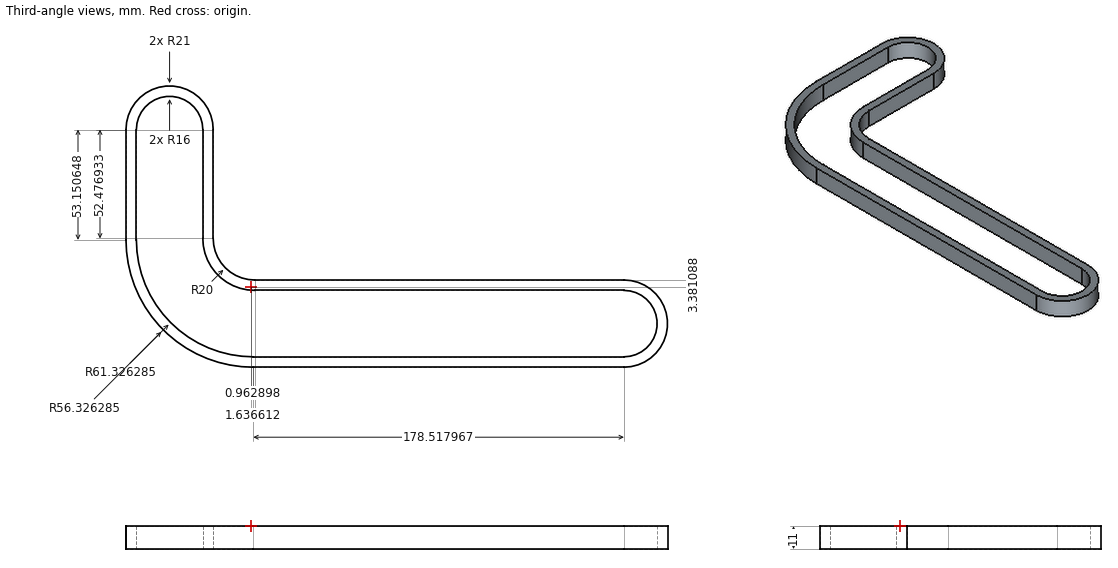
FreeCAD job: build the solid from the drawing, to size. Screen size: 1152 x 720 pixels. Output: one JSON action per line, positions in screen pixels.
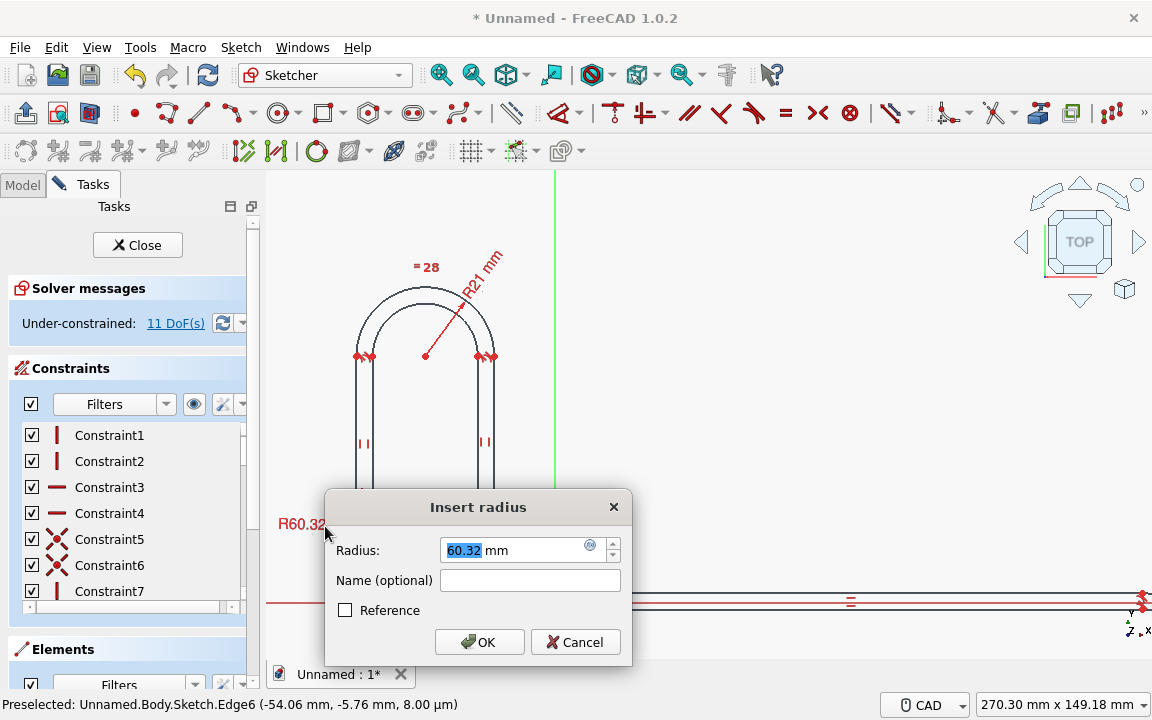
{"action": "type", "text": "61.326285"}
{"action": "key", "text": "Return"}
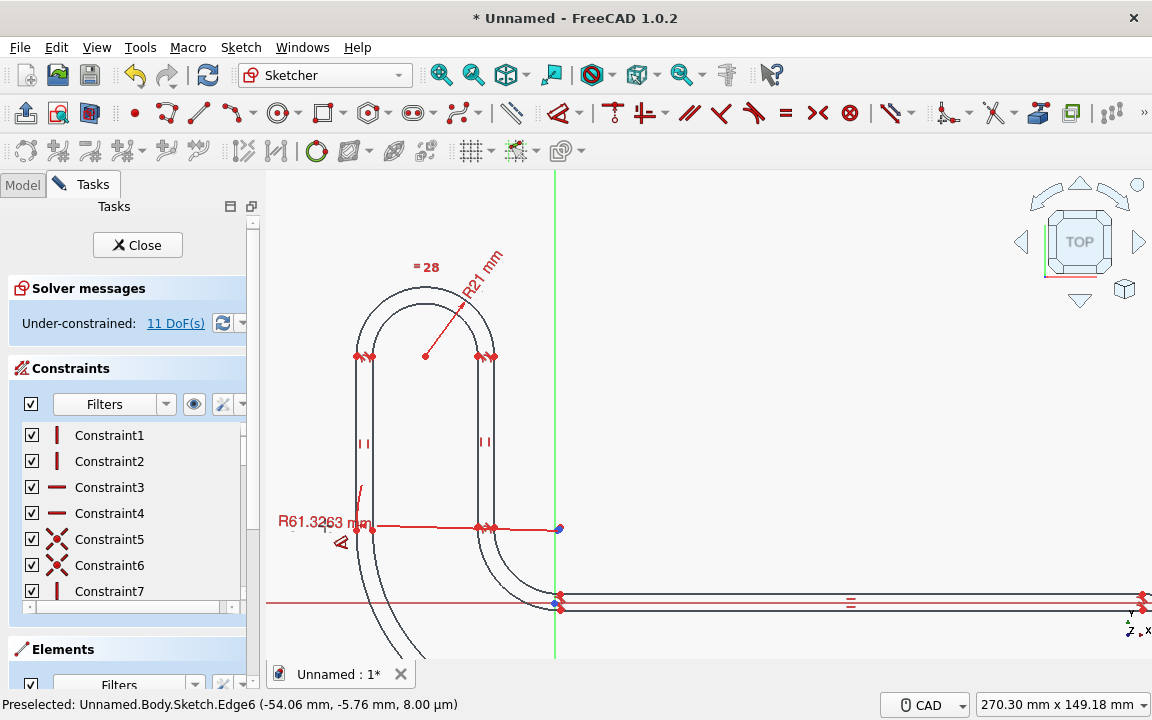
{"action": "left_click", "coordinate": [501, 558]}
{"action": "left_click", "coordinate": [473, 573]}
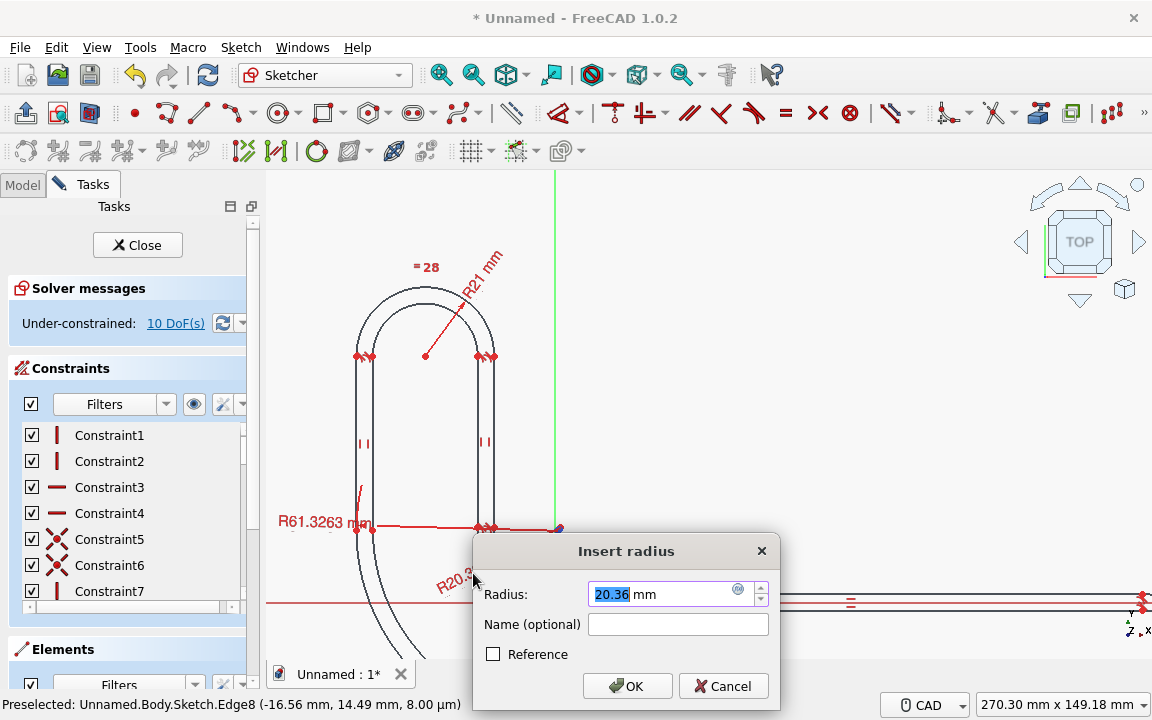
{"action": "type", "text": "20"}
{"action": "key", "text": "Return"}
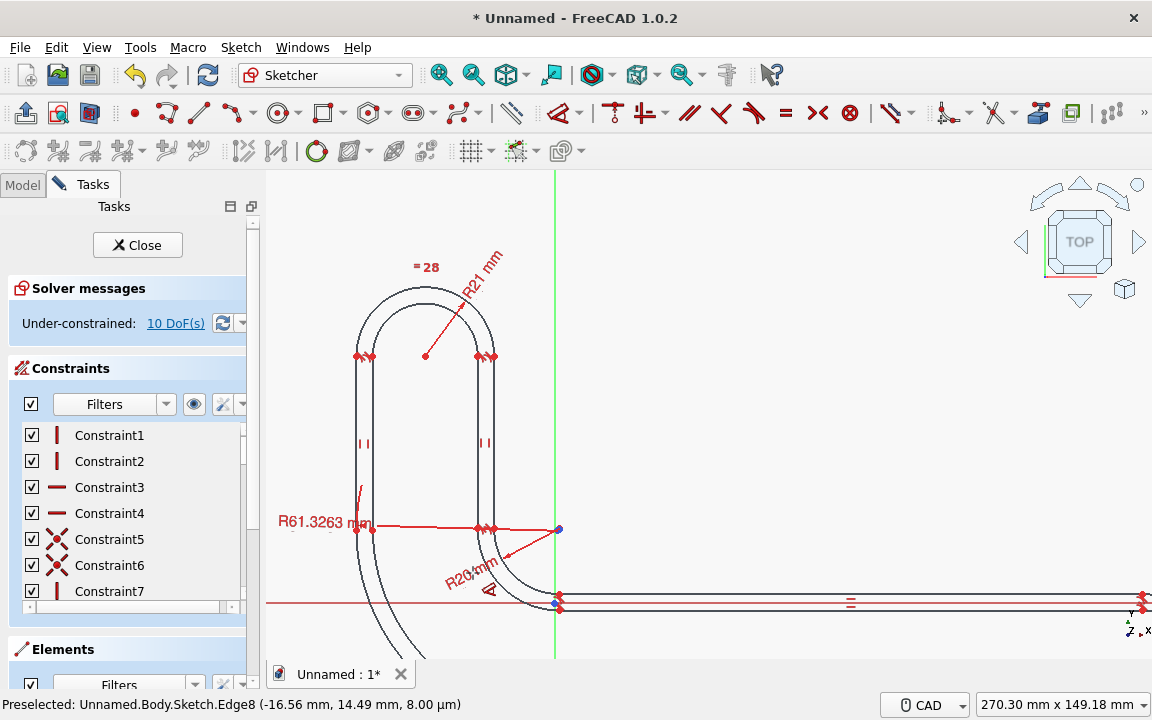
{"action": "left_click", "coordinate": [456, 314]}
{"action": "left_click", "coordinate": [501, 320]}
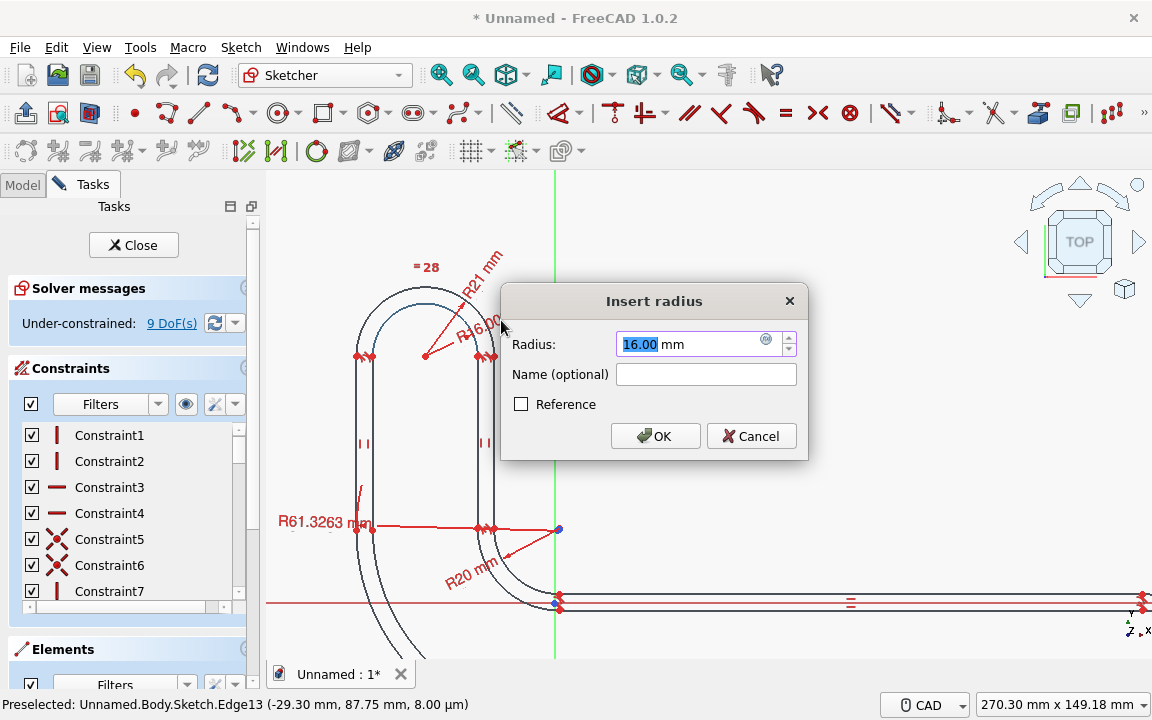
{"action": "type", "text": "16"}
{"action": "key", "text": "Return"}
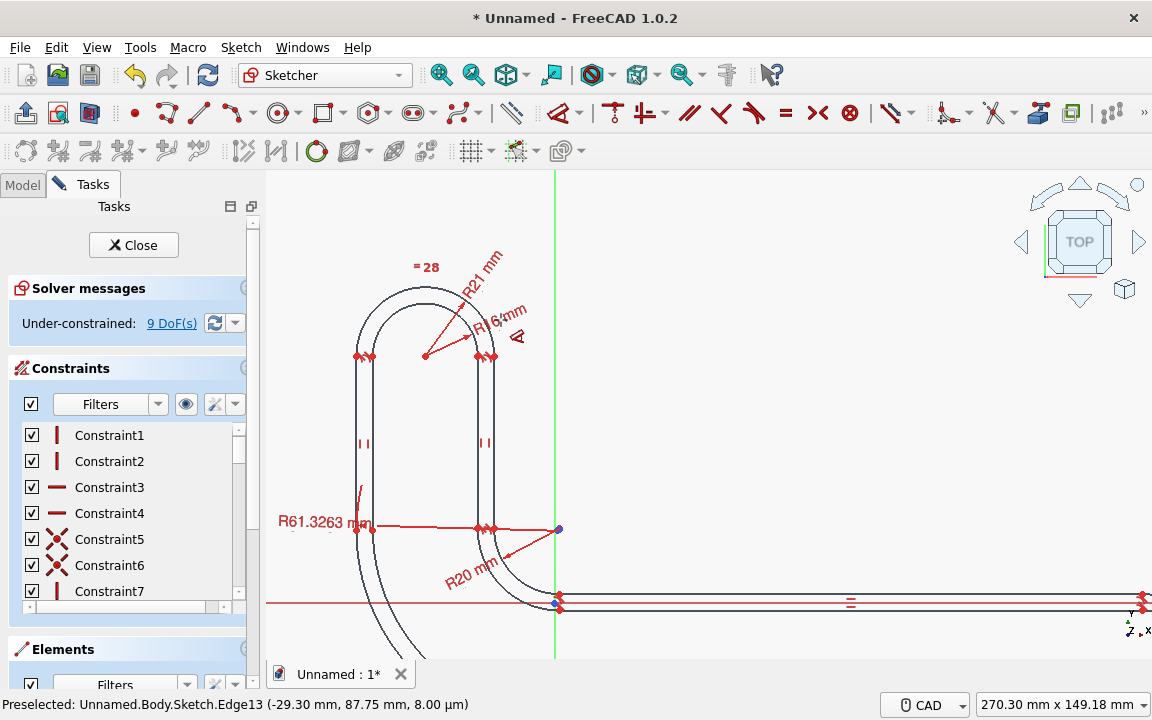
{"action": "scroll", "coordinate": [393, 614], "scroll_direction": "up", "scroll_amount": 2}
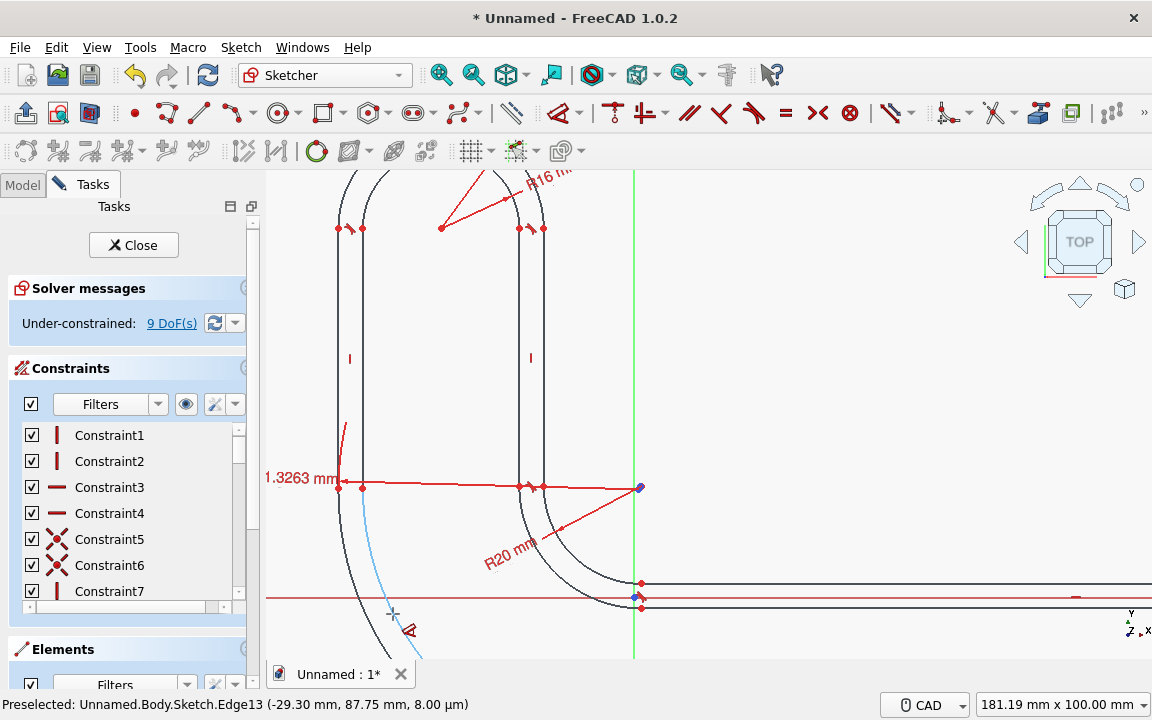
{"action": "left_click", "coordinate": [393, 613]}
{"action": "left_click", "coordinate": [500, 211]}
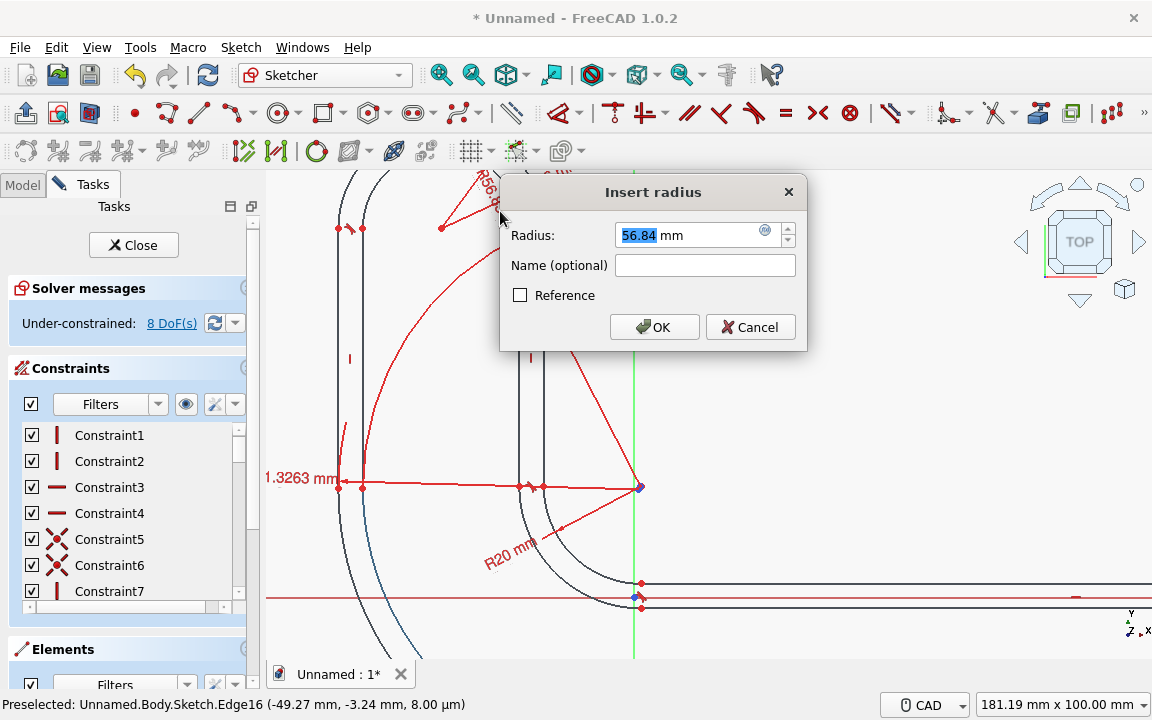
{"action": "type", "text": "56.326285"}
{"action": "key", "text": "Return"}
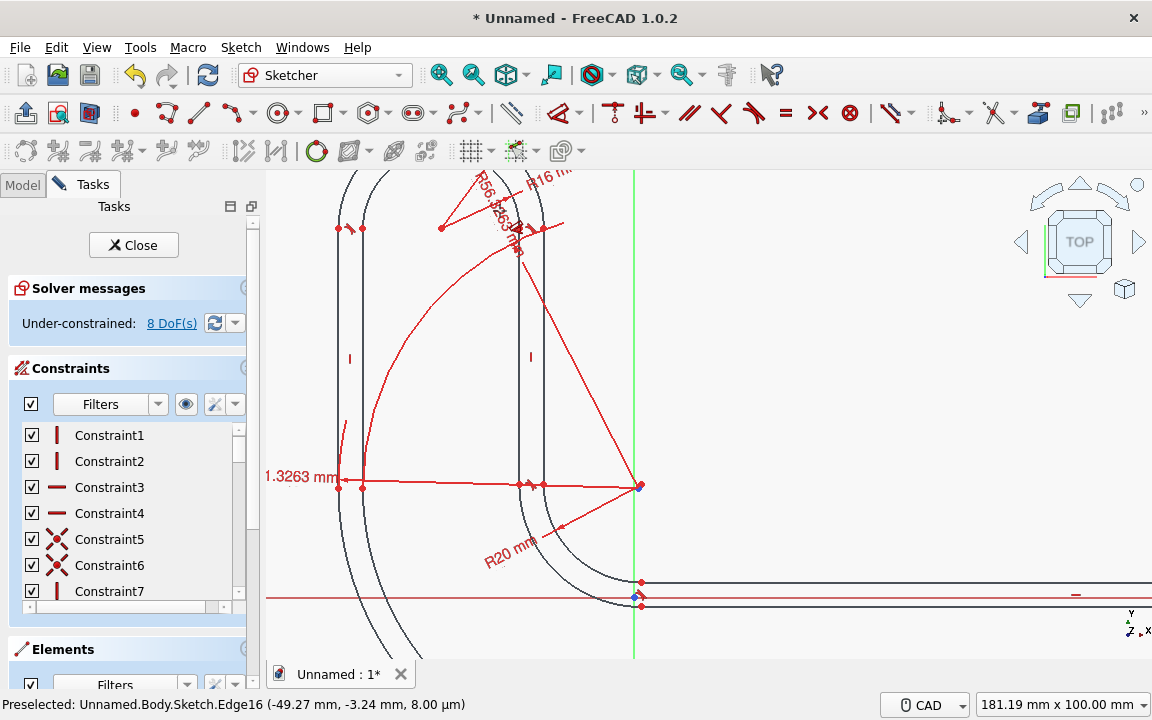
{"action": "left_click", "coordinate": [544, 408]}
{"action": "left_click", "coordinate": [578, 357]}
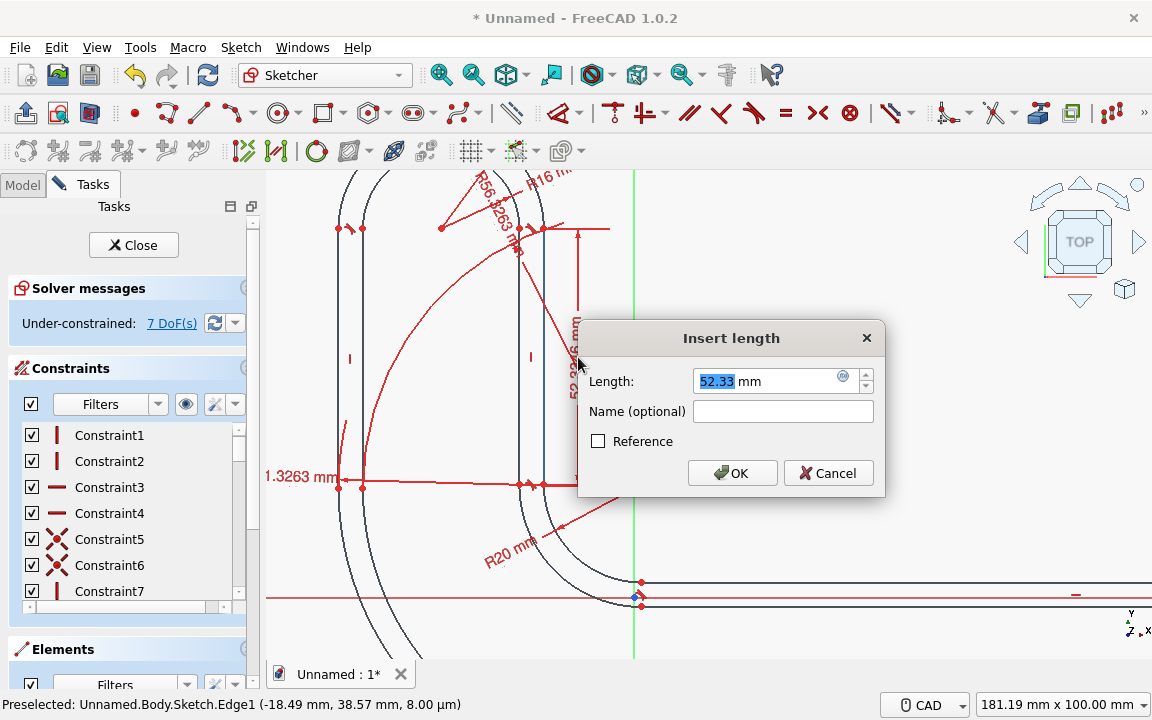
{"action": "type", "text": "52.476933"}
{"action": "key", "text": "Return"}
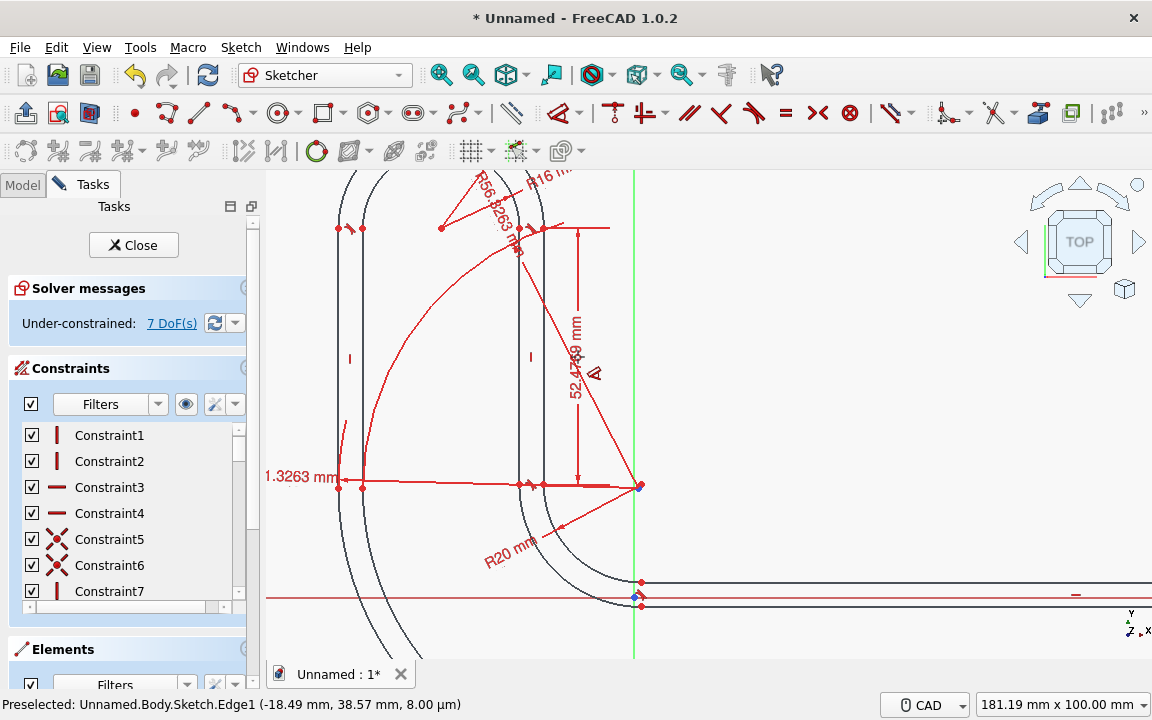
{"action": "left_click", "coordinate": [338, 306]}
{"action": "left_click", "coordinate": [304, 358]}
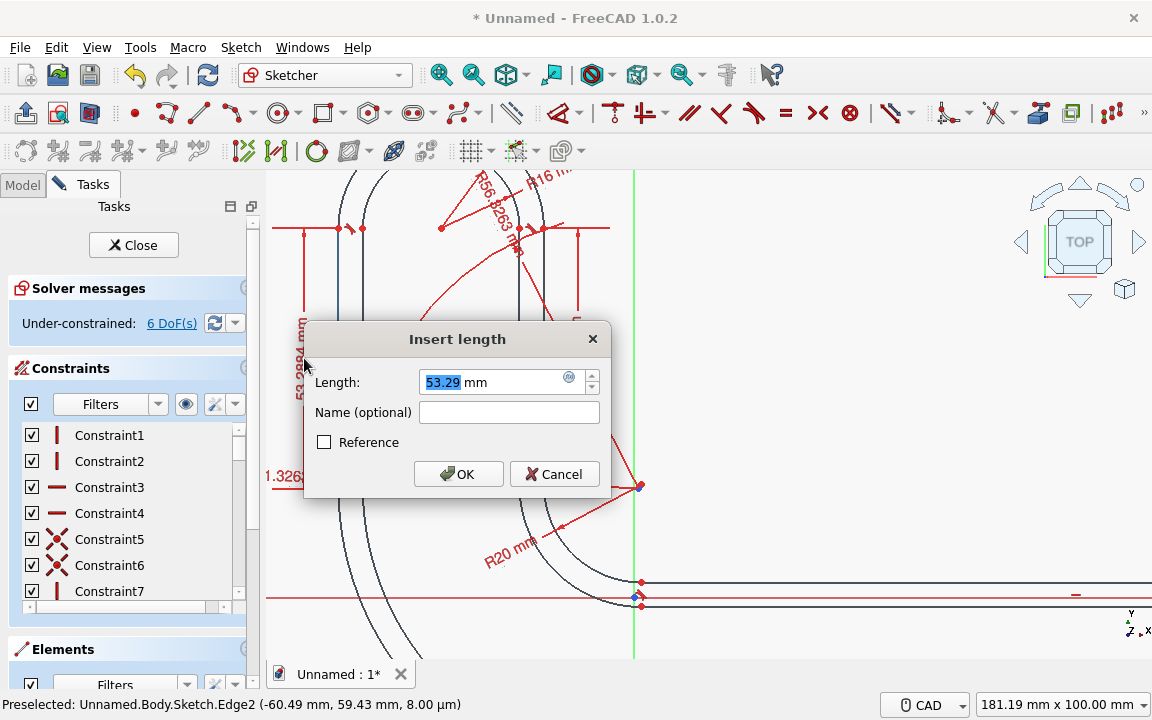
{"action": "type", "text": "53.150648"}
{"action": "key", "text": "Return"}